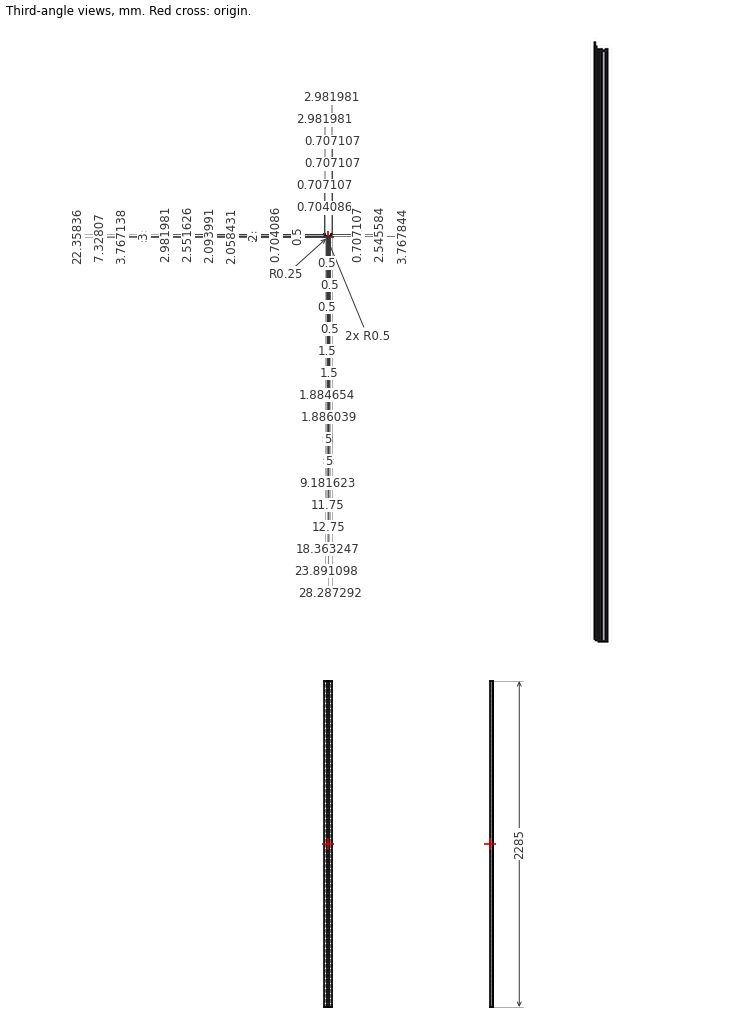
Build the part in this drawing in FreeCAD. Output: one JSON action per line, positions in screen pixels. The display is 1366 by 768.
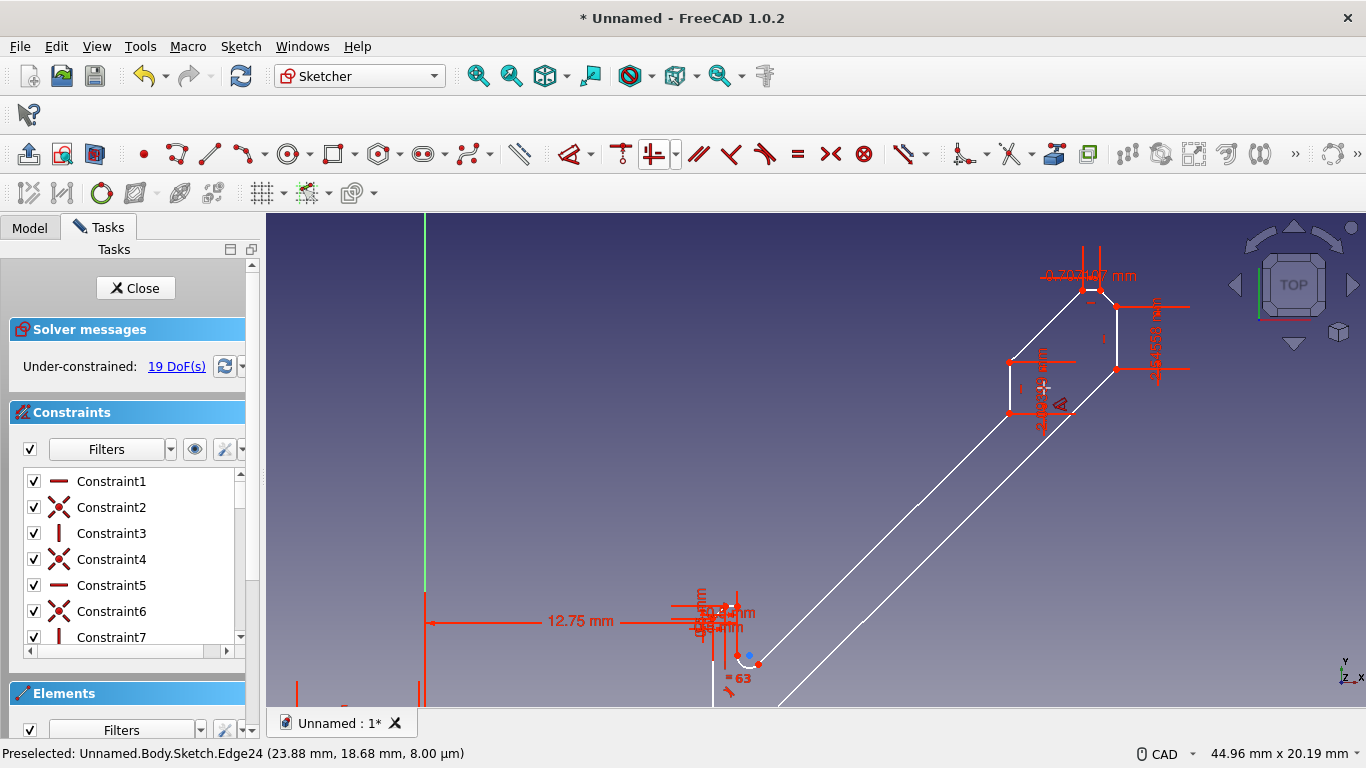
{"action": "left_click", "coordinate": [737, 641]}
{"action": "left_click", "coordinate": [795, 648]}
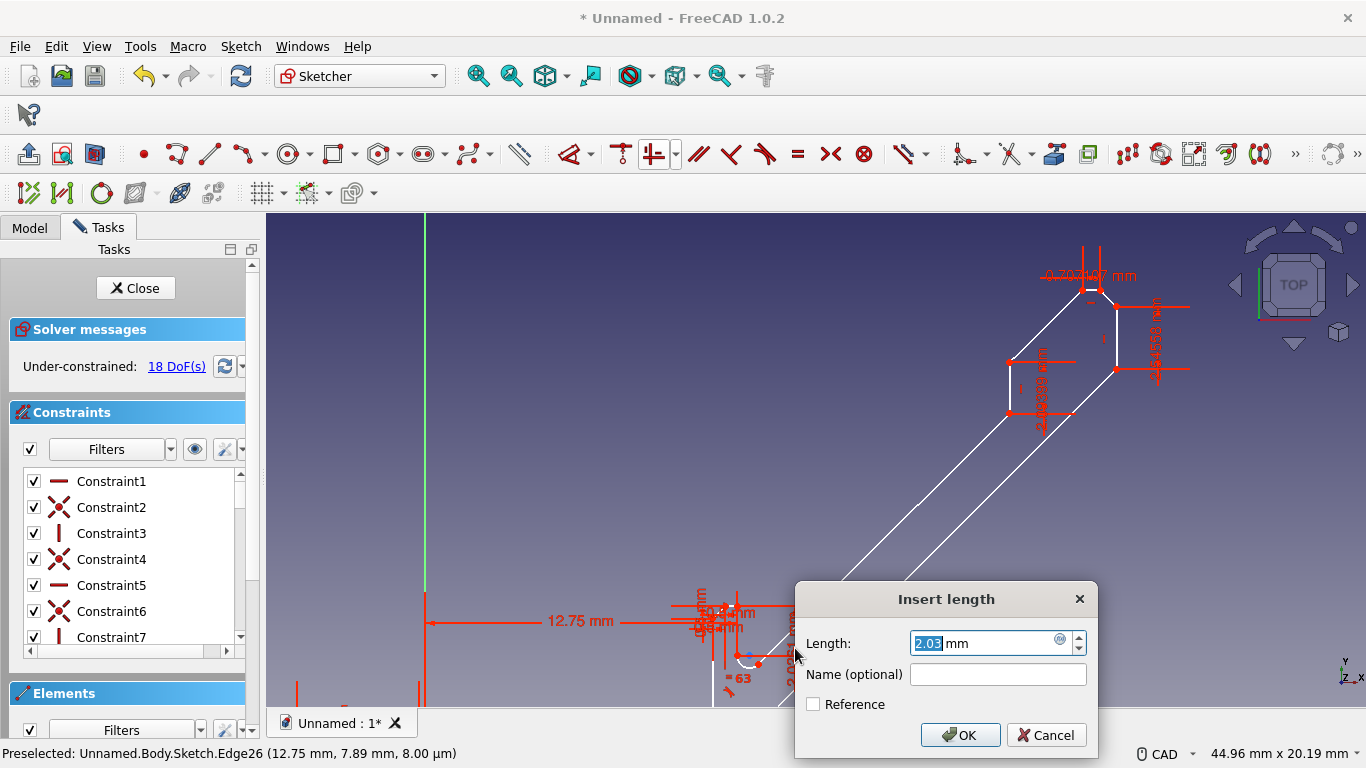
{"action": "type", "text": "2.058431"}
{"action": "key", "text": "Return"}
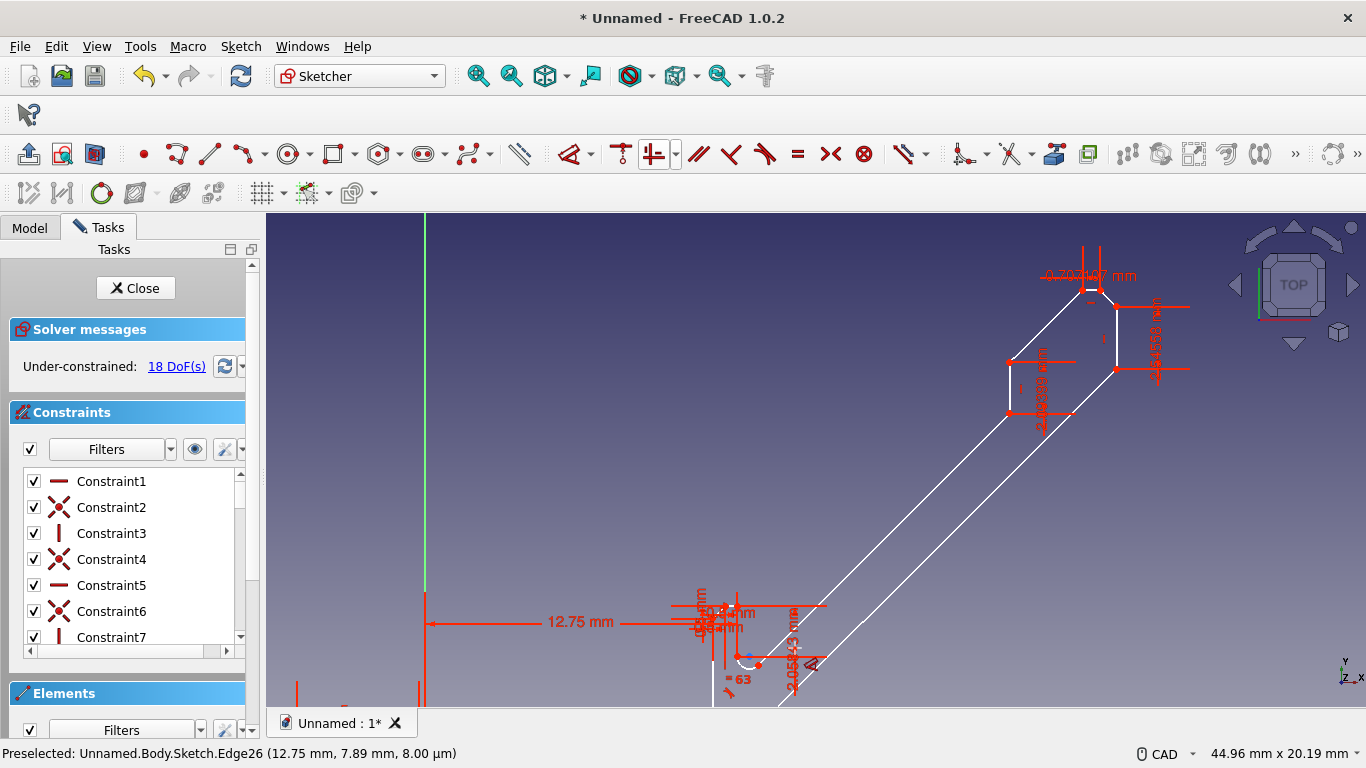
{"action": "left_click", "coordinate": [713, 646]}
{"action": "left_click", "coordinate": [679, 663]}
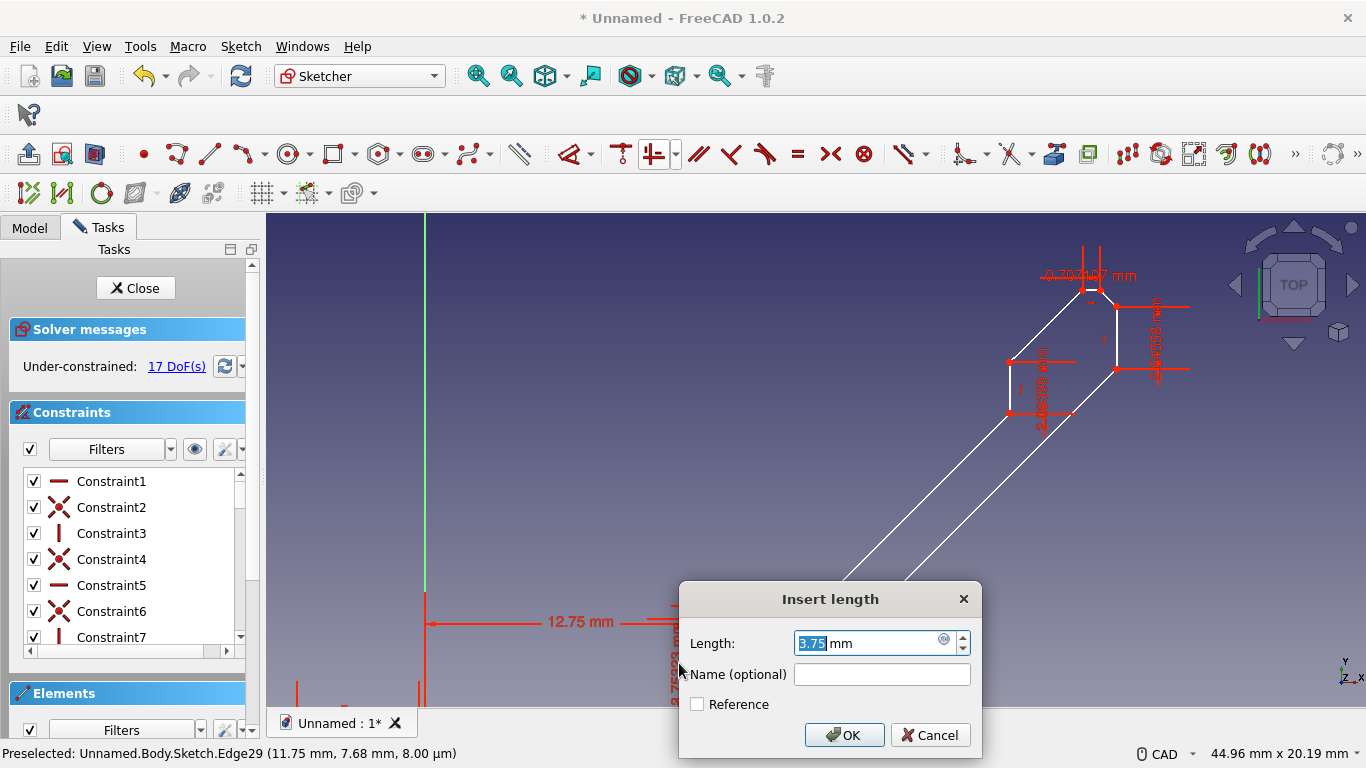
{"action": "type", "text": "3.767844"}
{"action": "key", "text": "Return"}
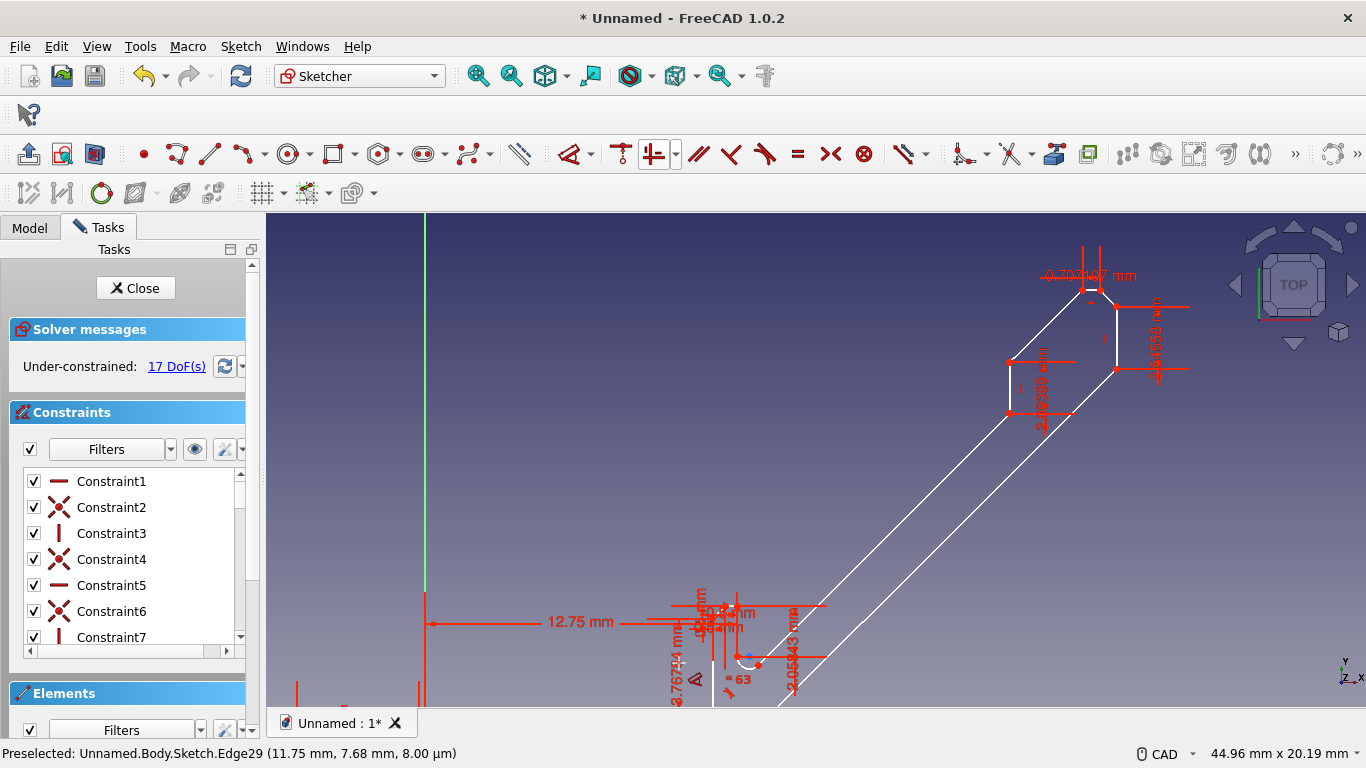
{"action": "scroll", "coordinate": [1010, 377], "scroll_direction": "down", "scroll_amount": 4}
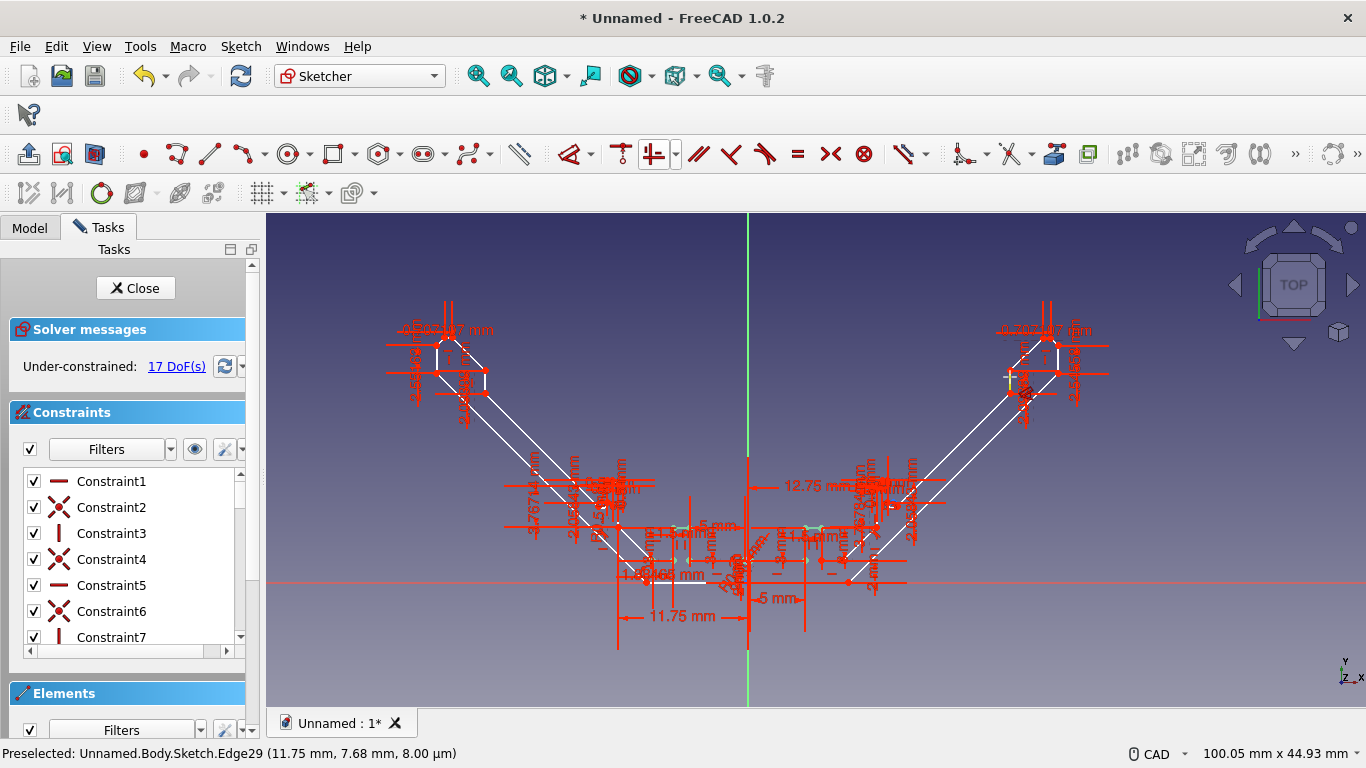
{"action": "scroll", "coordinate": [837, 561], "scroll_direction": "up", "scroll_amount": 4}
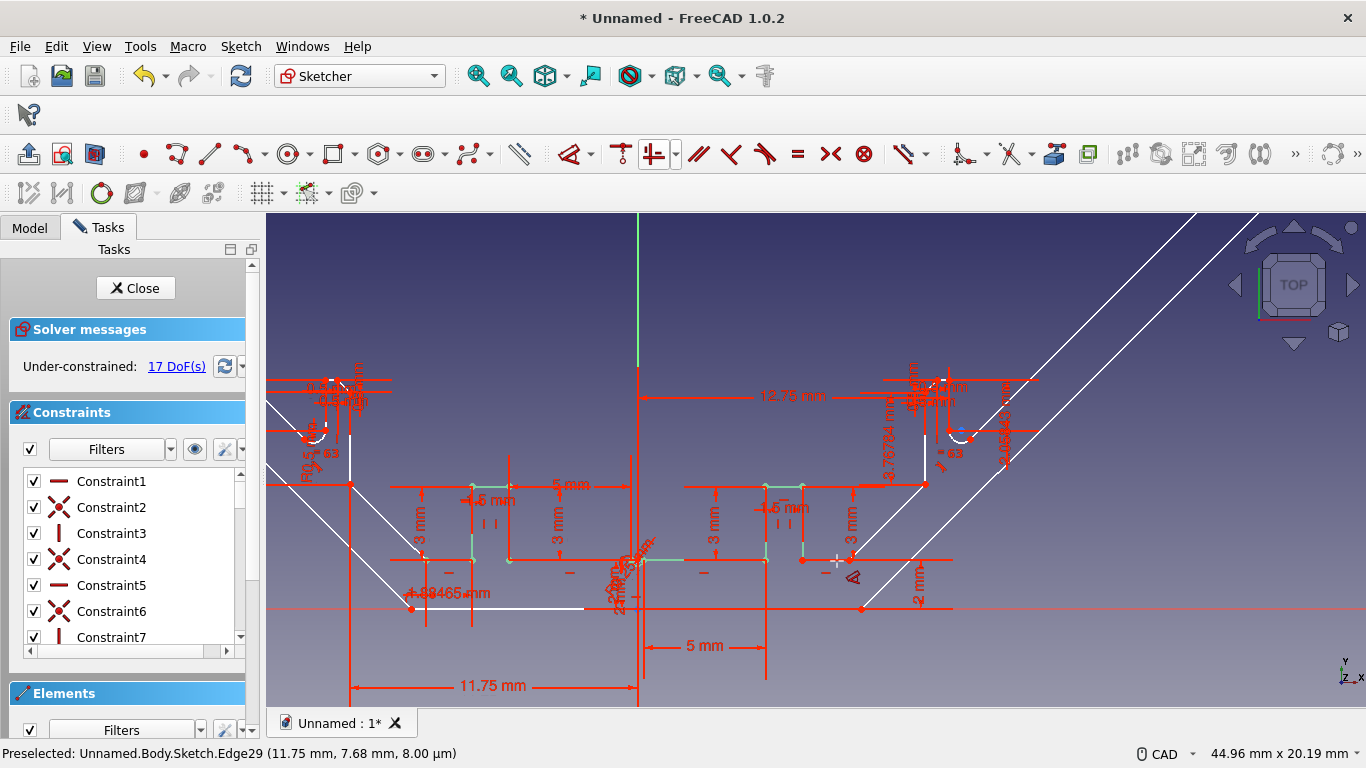
{"action": "left_click", "coordinate": [836, 560]}
{"action": "left_click", "coordinate": [826, 594]}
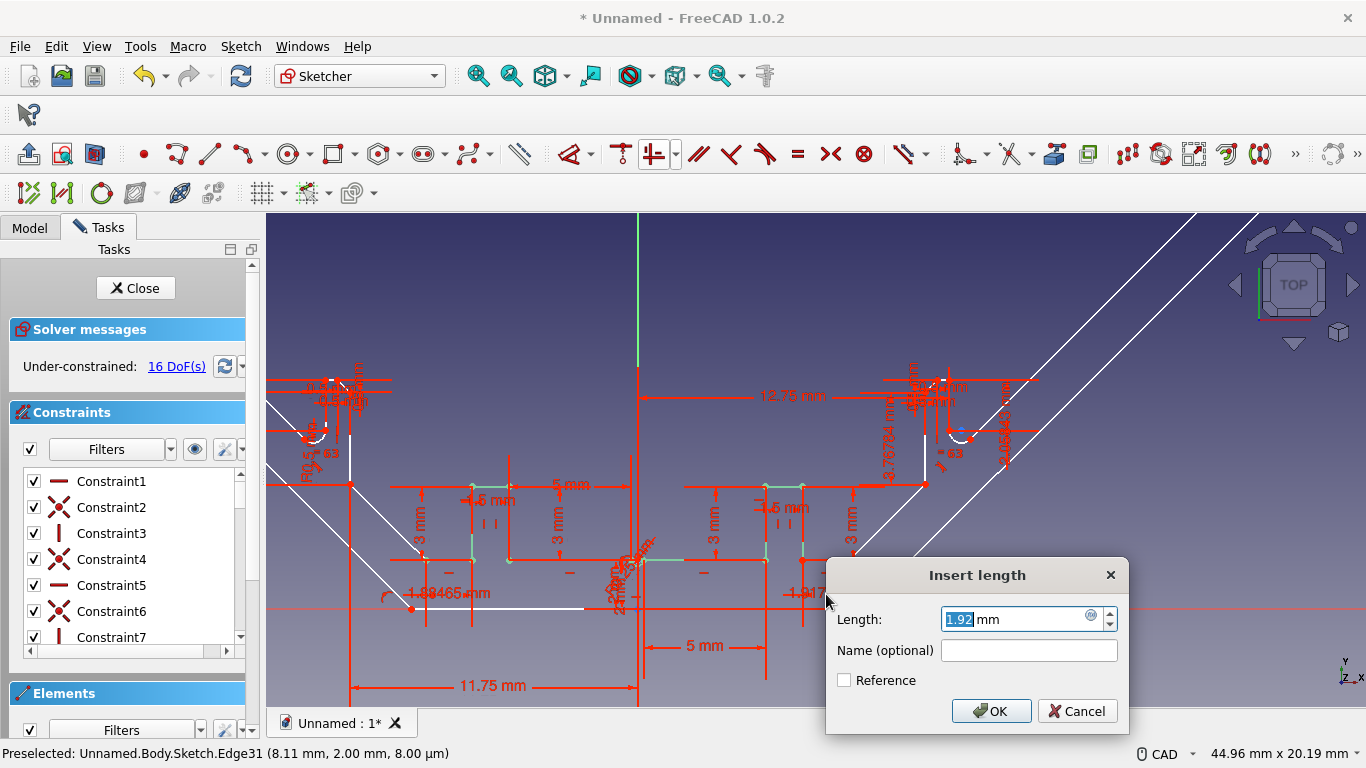
{"action": "type", "text": "1.886039"}
{"action": "key", "text": "Return"}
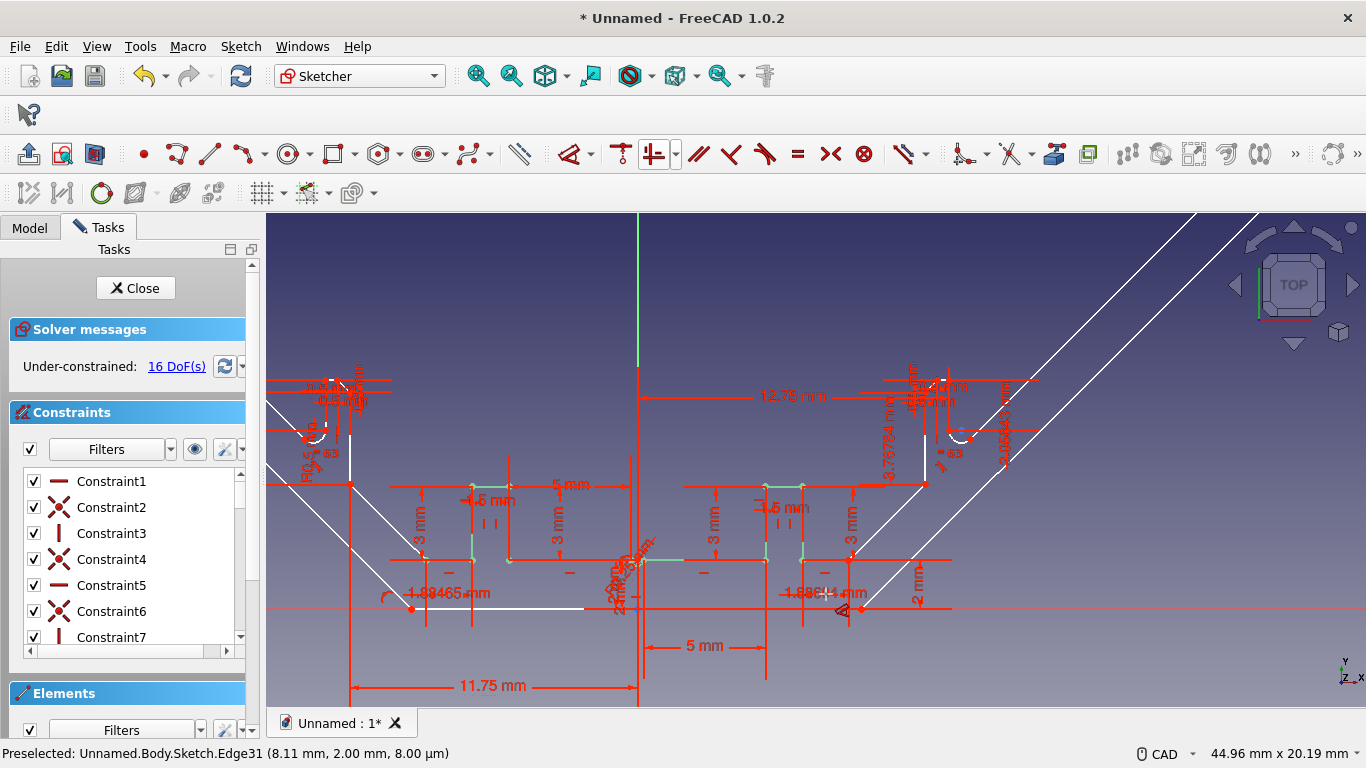
{"action": "left_click", "coordinate": [326, 431]}
{"action": "left_click", "coordinate": [672, 479]}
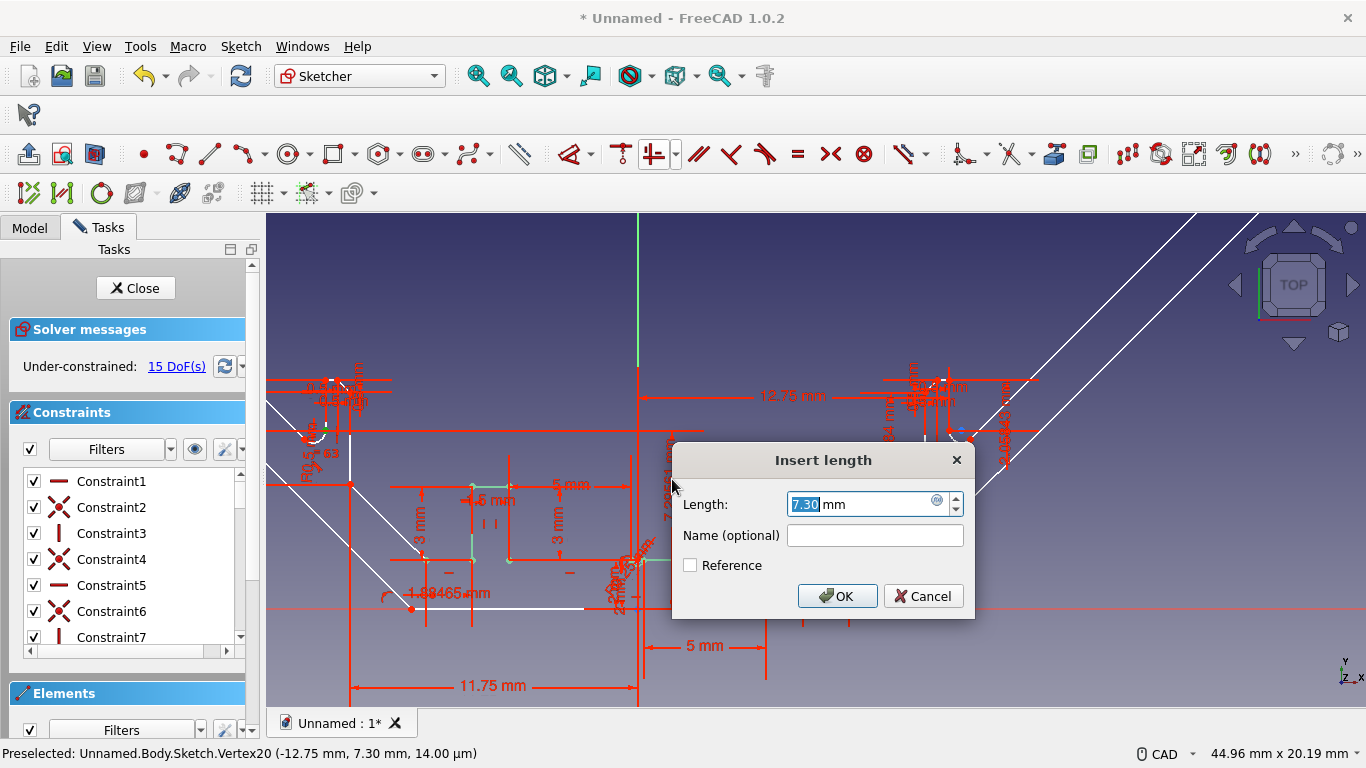
{"action": "type", "text": "7.32807"}
{"action": "key", "text": "Return"}